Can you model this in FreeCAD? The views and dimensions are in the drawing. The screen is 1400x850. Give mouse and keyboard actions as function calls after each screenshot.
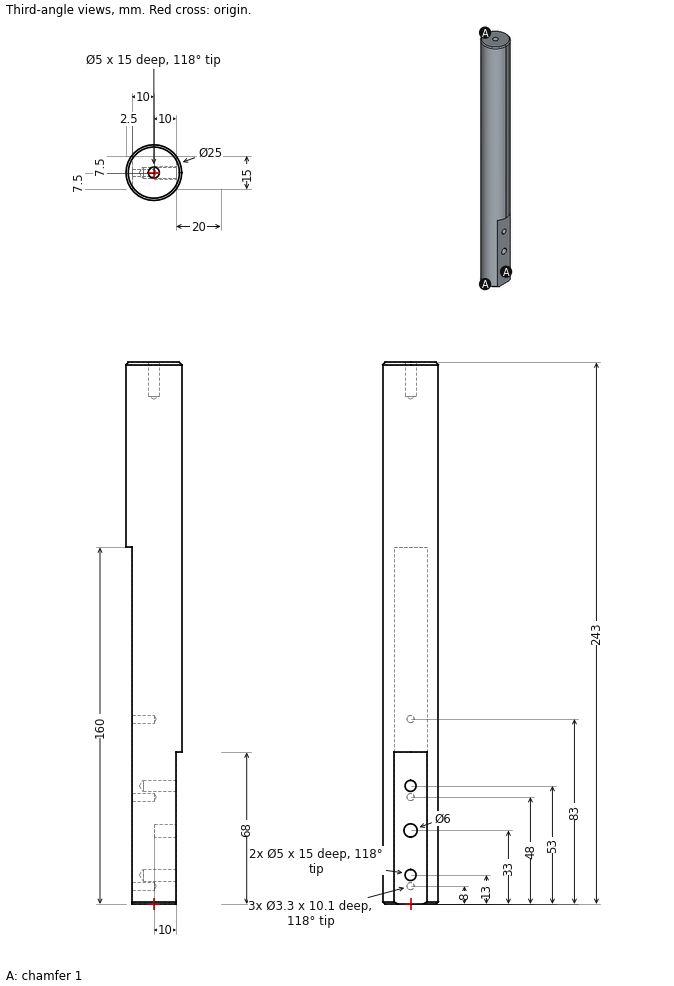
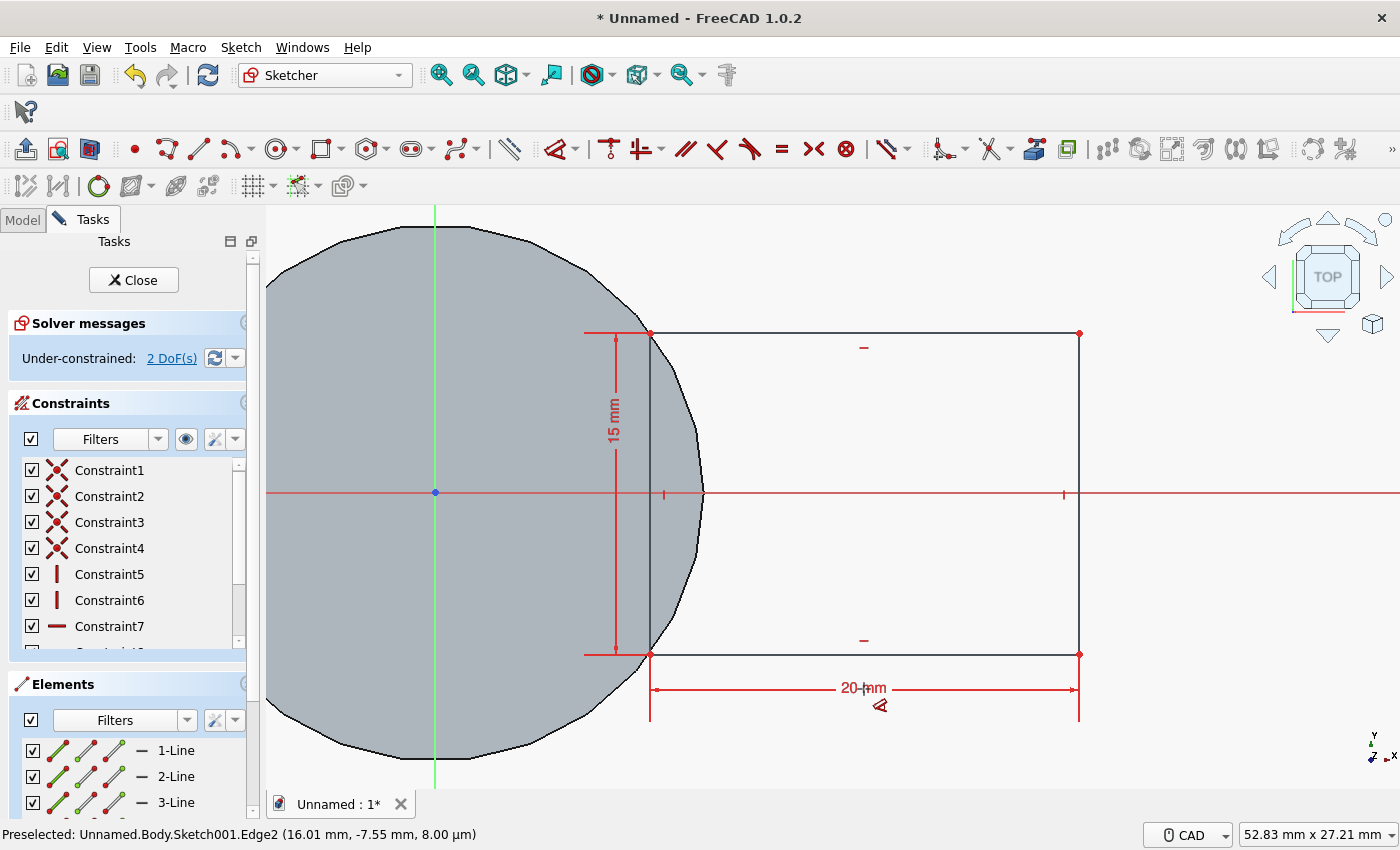
click(650, 333)
click(543, 299)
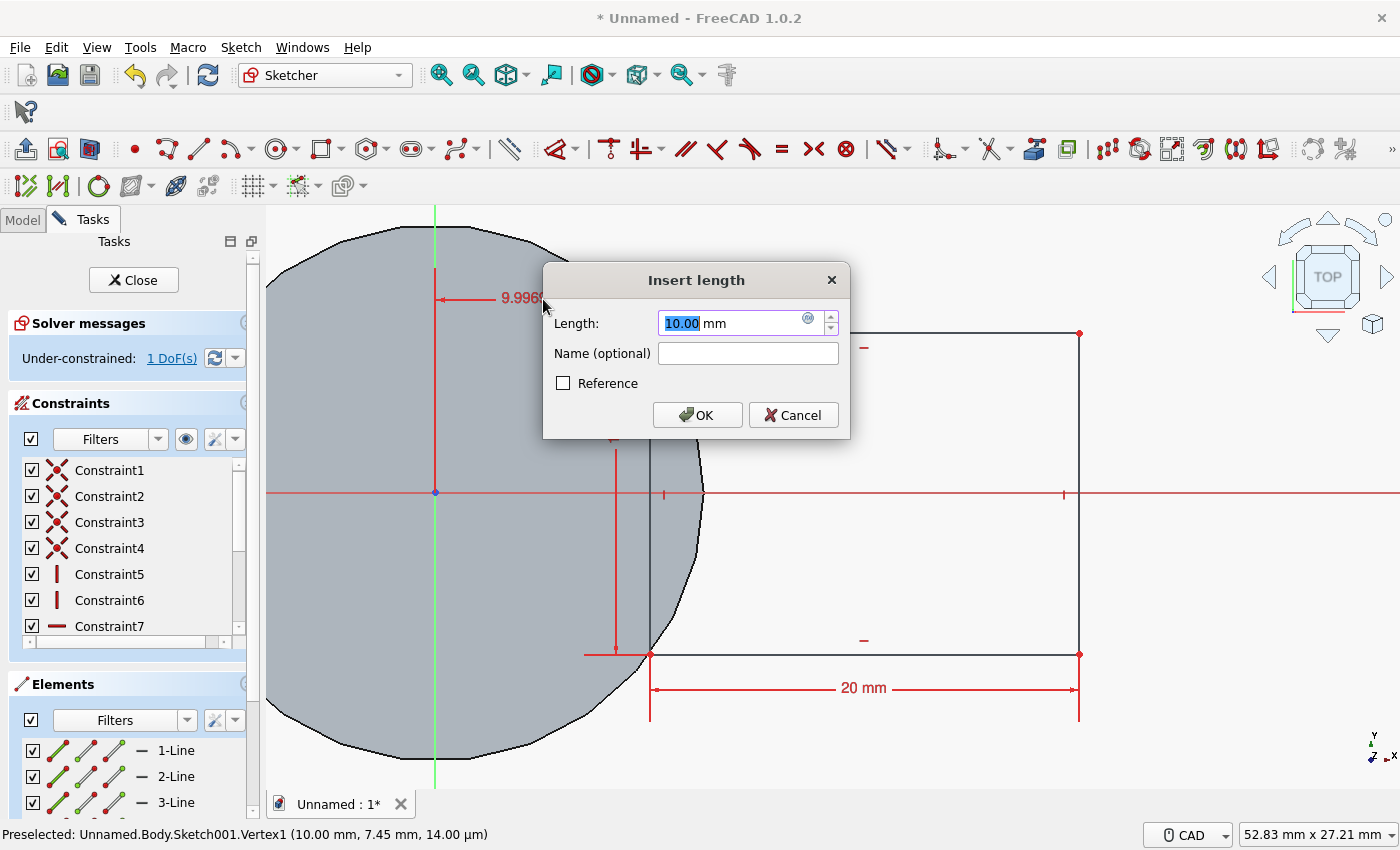
text(10)
key(Return)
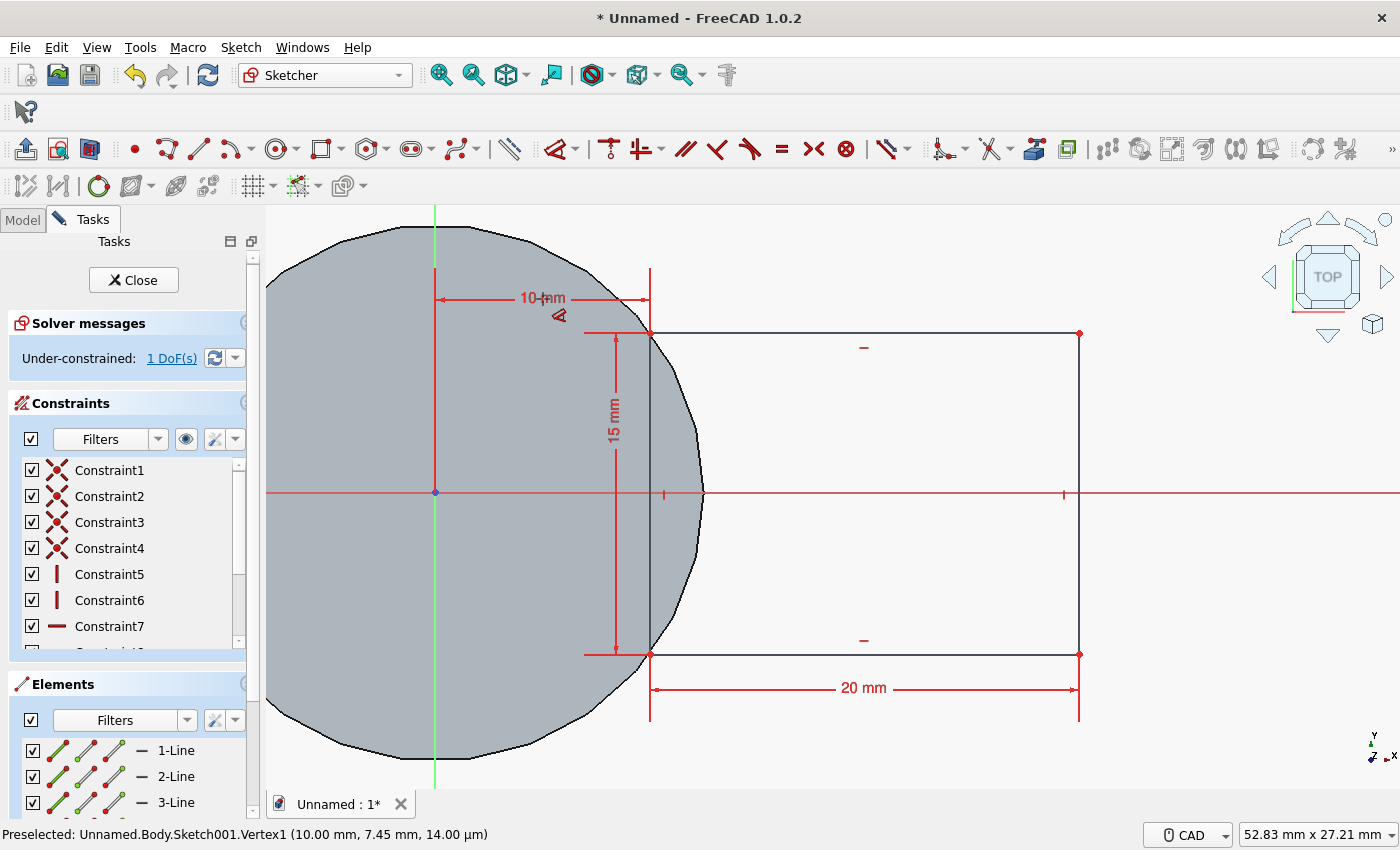
click(650, 333)
click(401, 413)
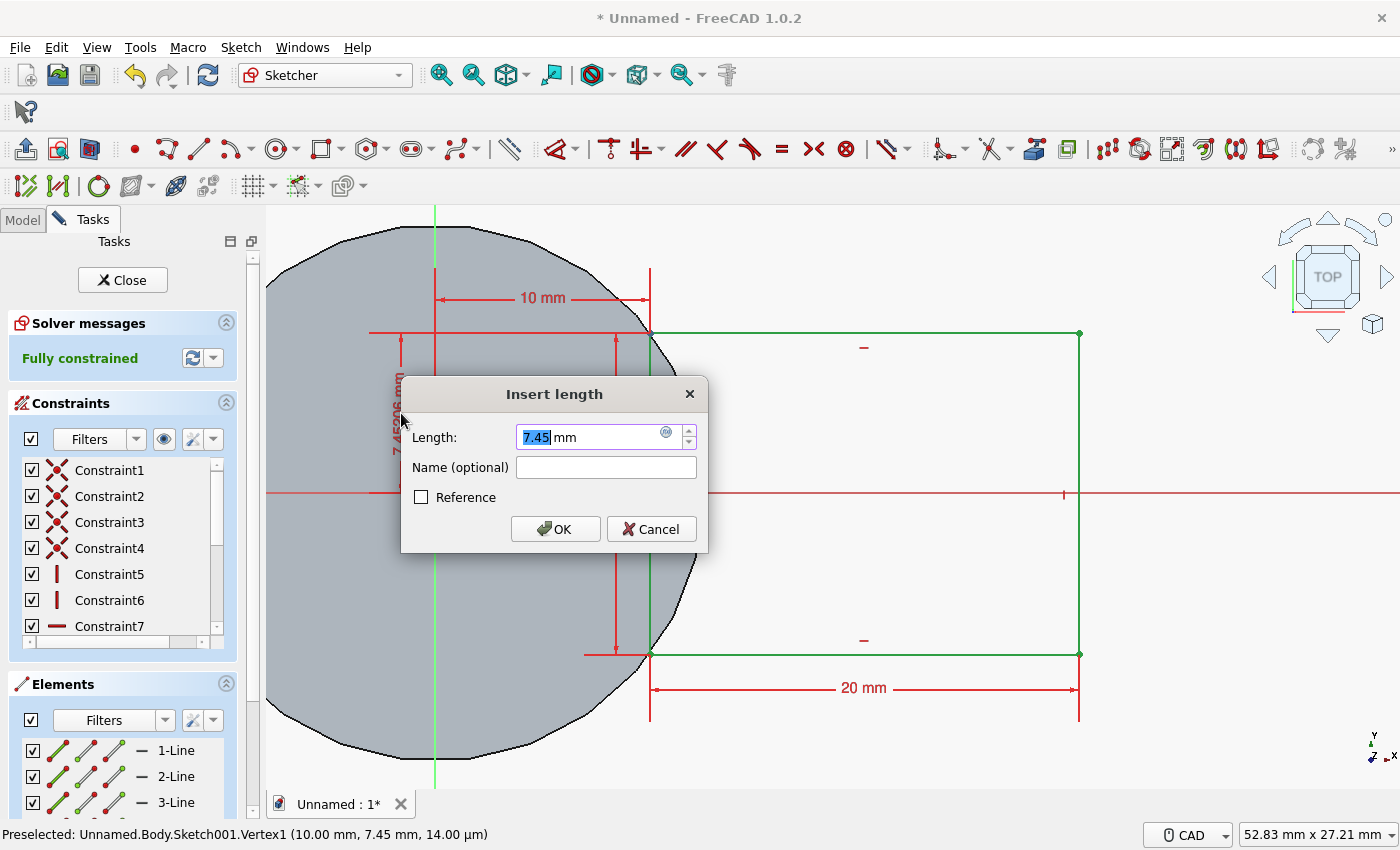
text(7.5)
key(Return)
key(Escape)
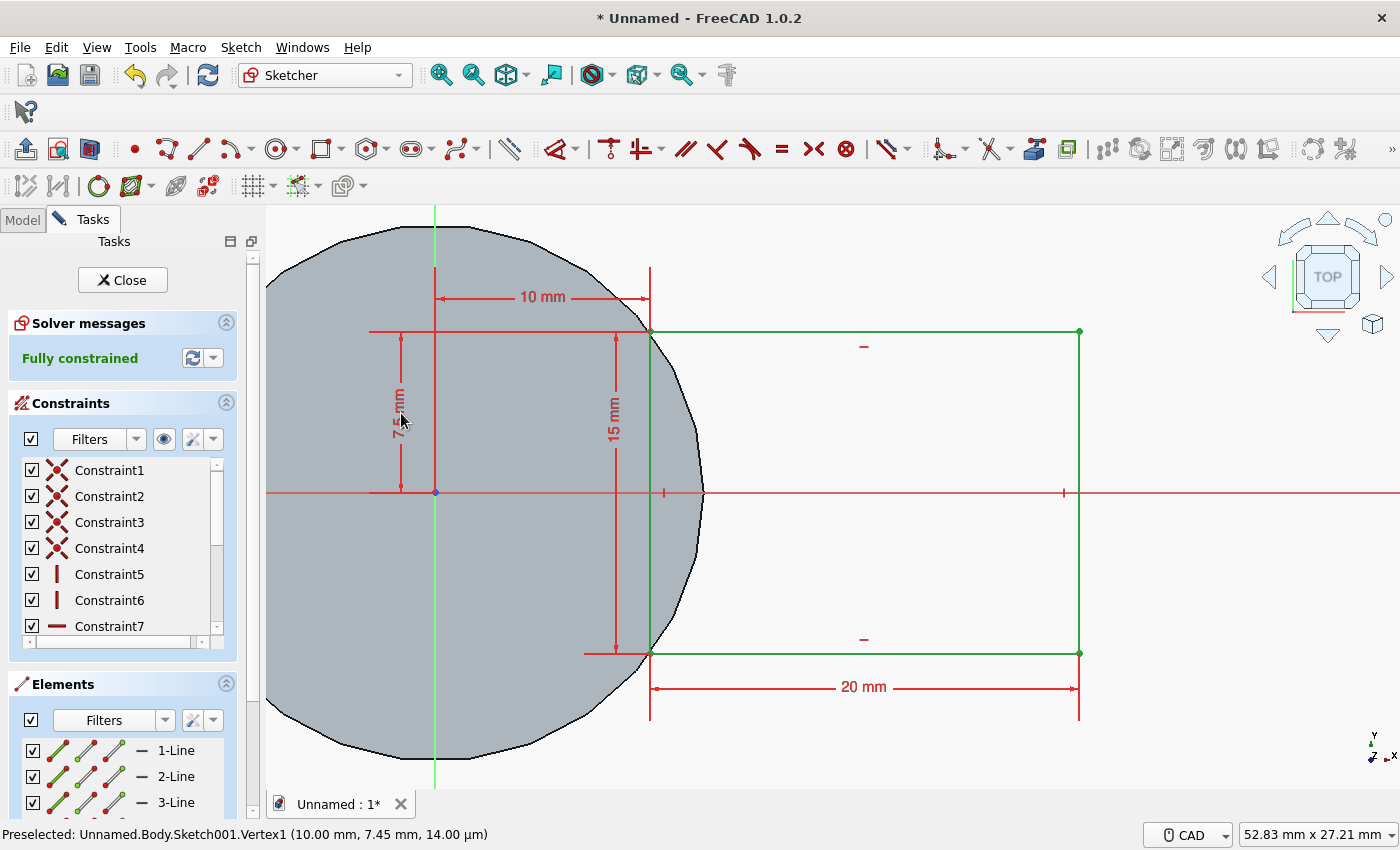
click(123, 280)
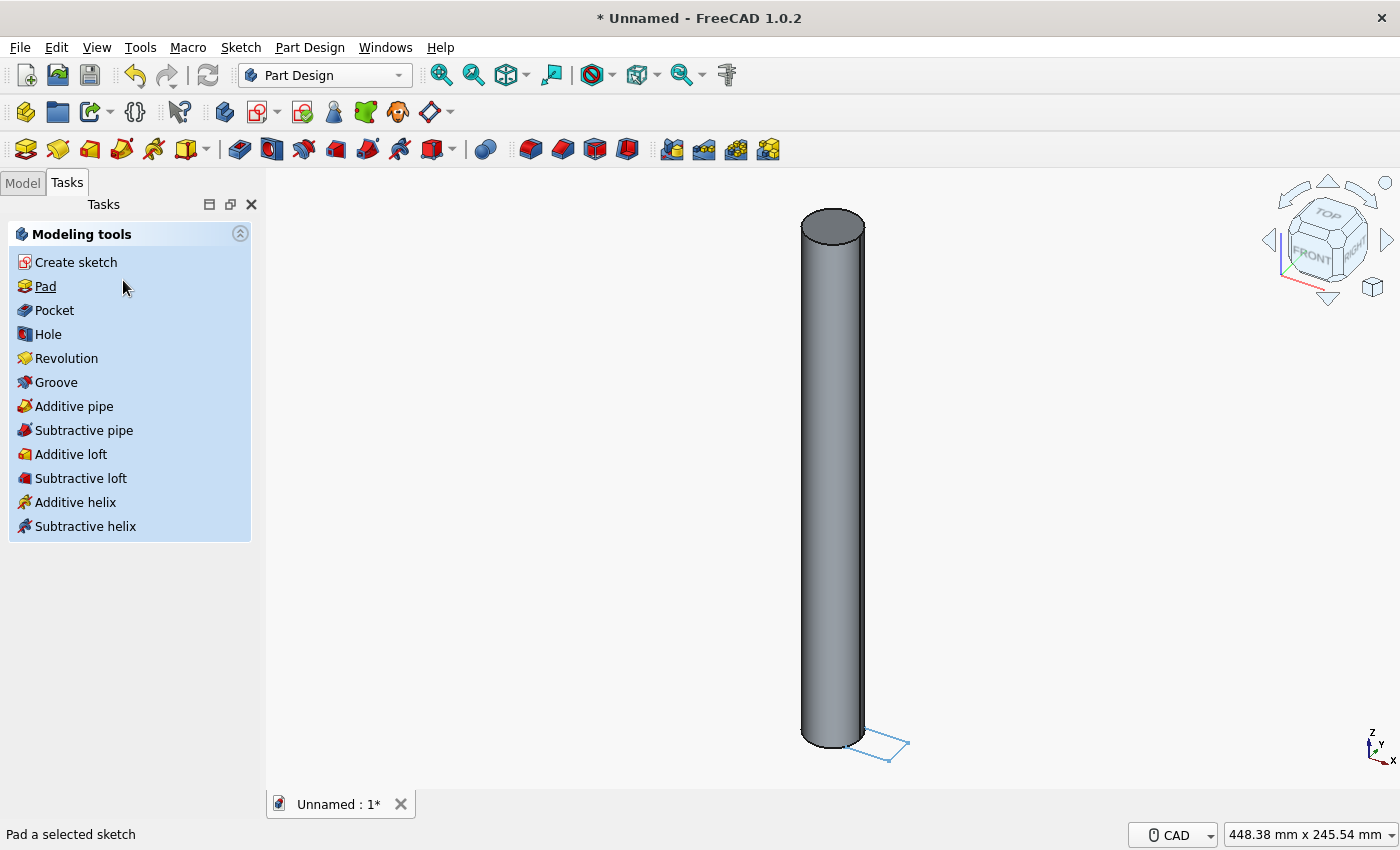
click(240, 150)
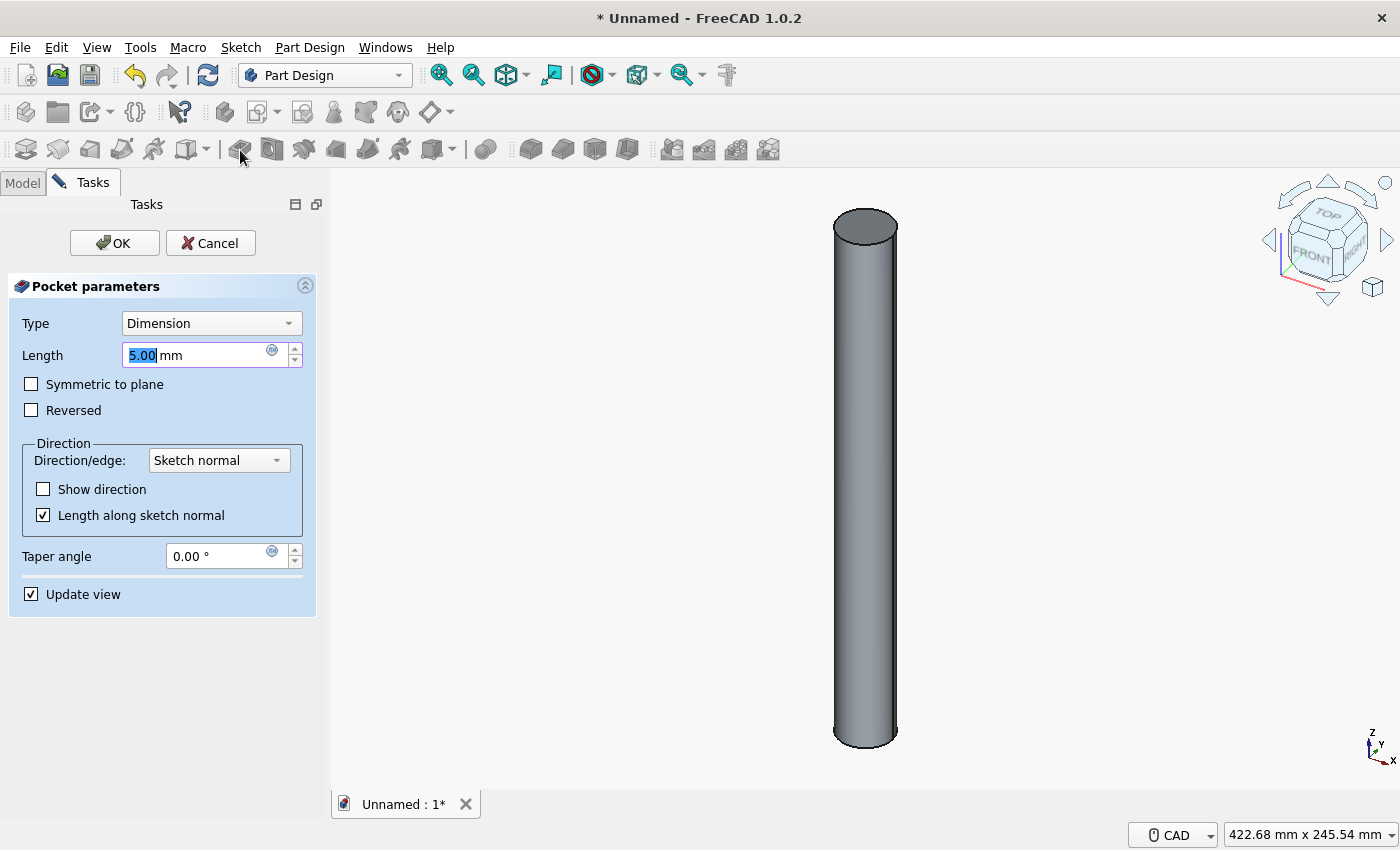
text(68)
key(Tab)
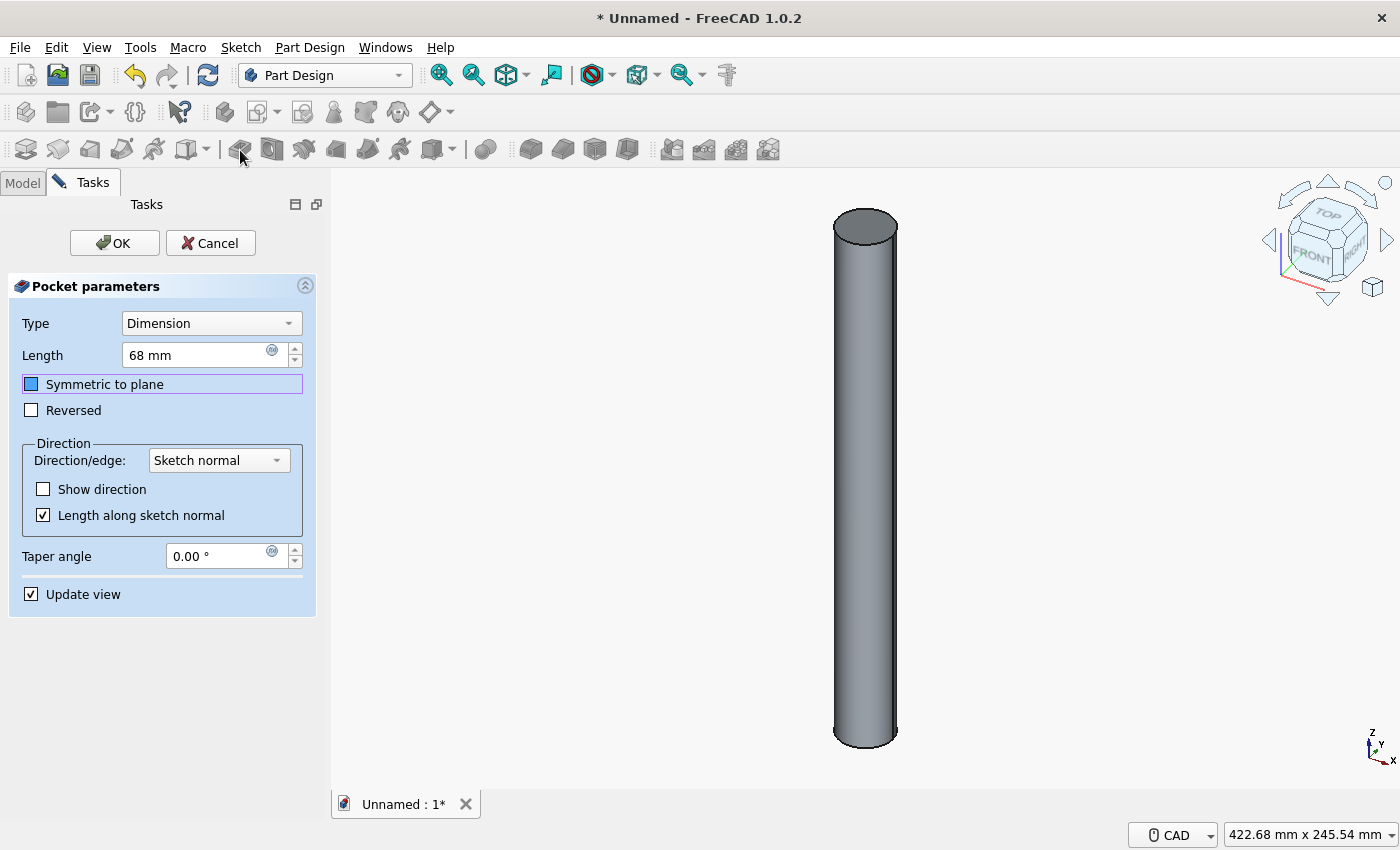
click(30, 410)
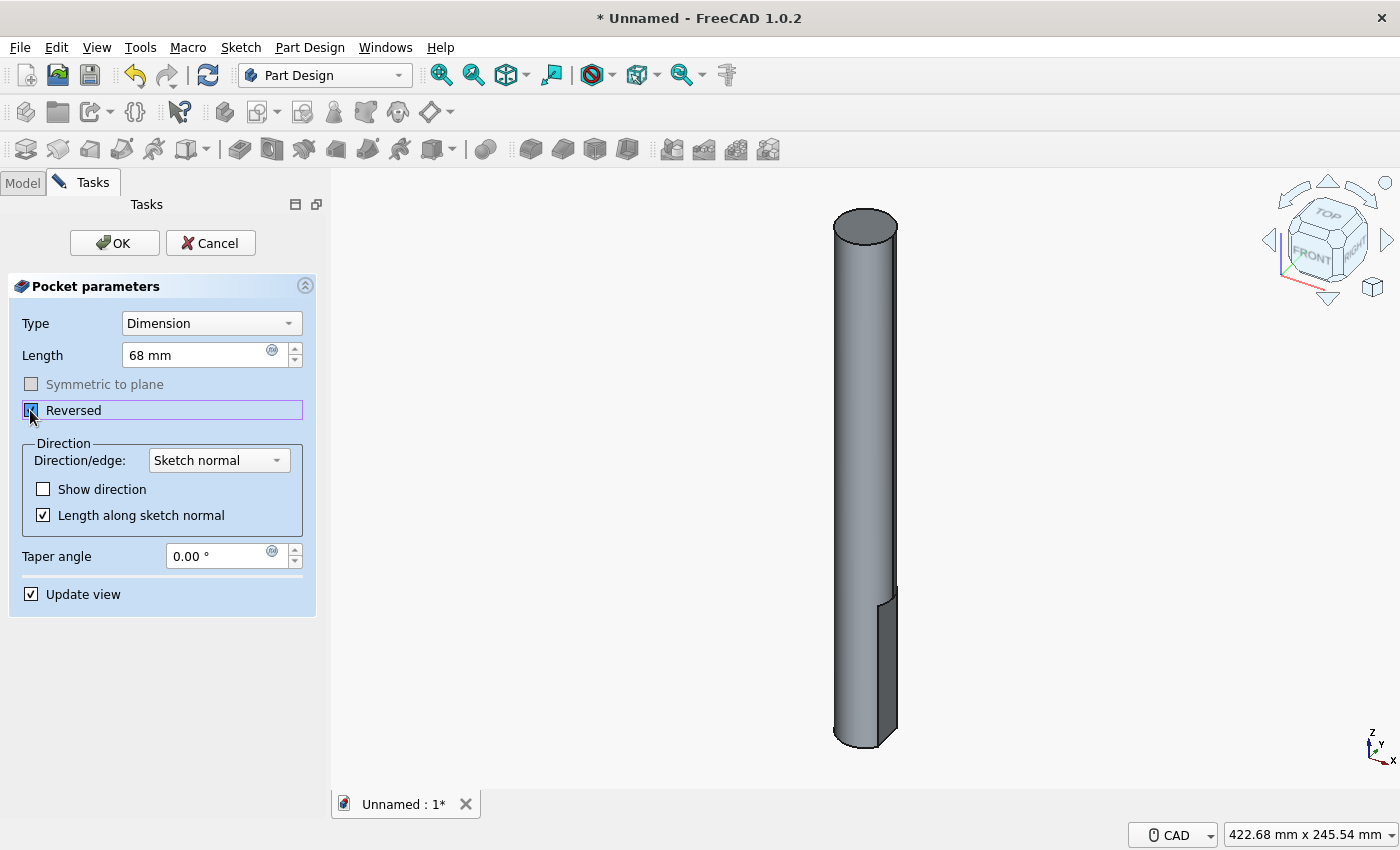
click(115, 243)